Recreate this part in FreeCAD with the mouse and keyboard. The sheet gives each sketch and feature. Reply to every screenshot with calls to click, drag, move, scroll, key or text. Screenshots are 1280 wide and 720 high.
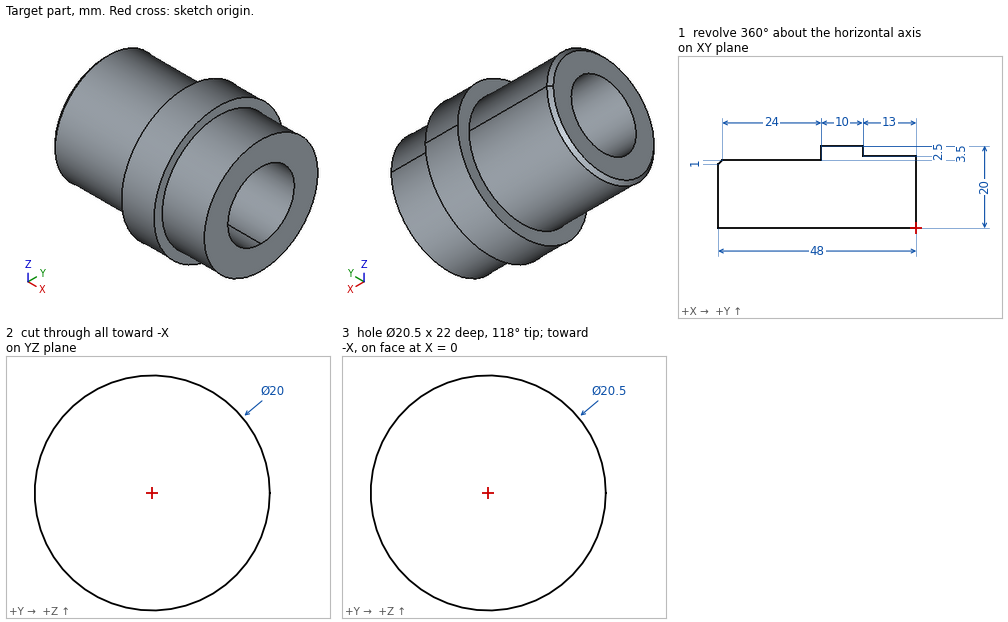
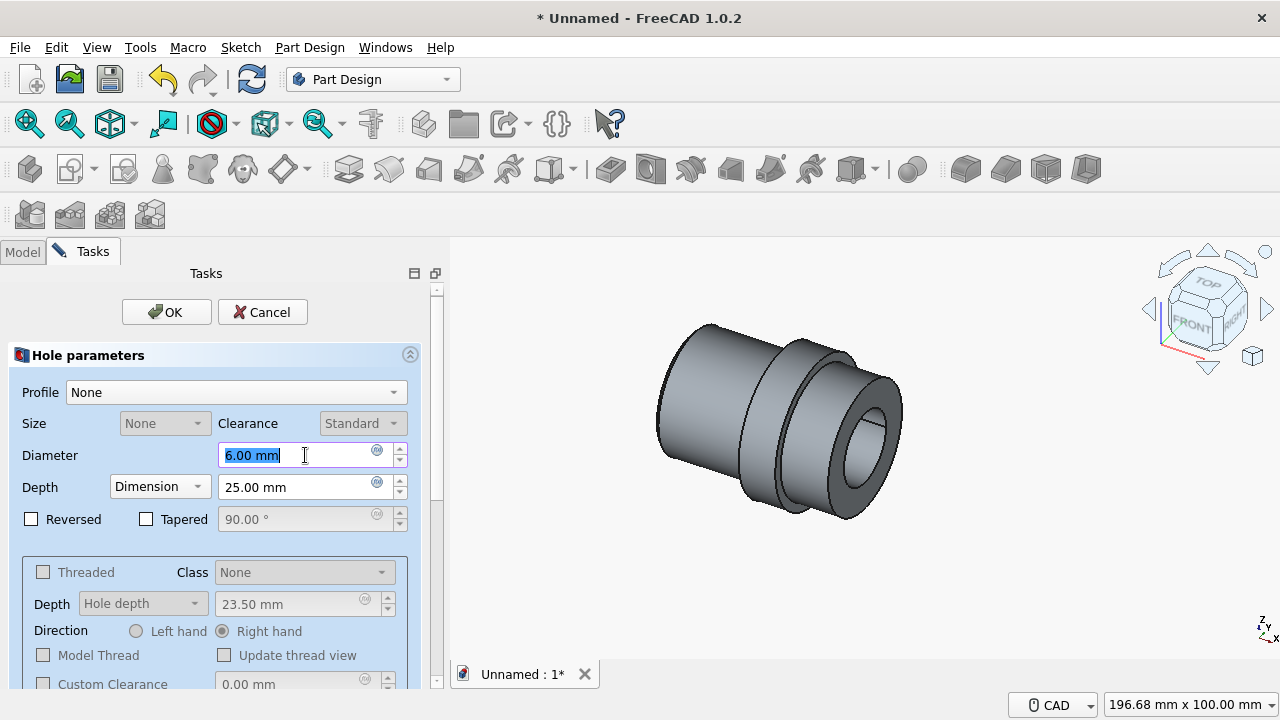
text(20.5)
key(Tab)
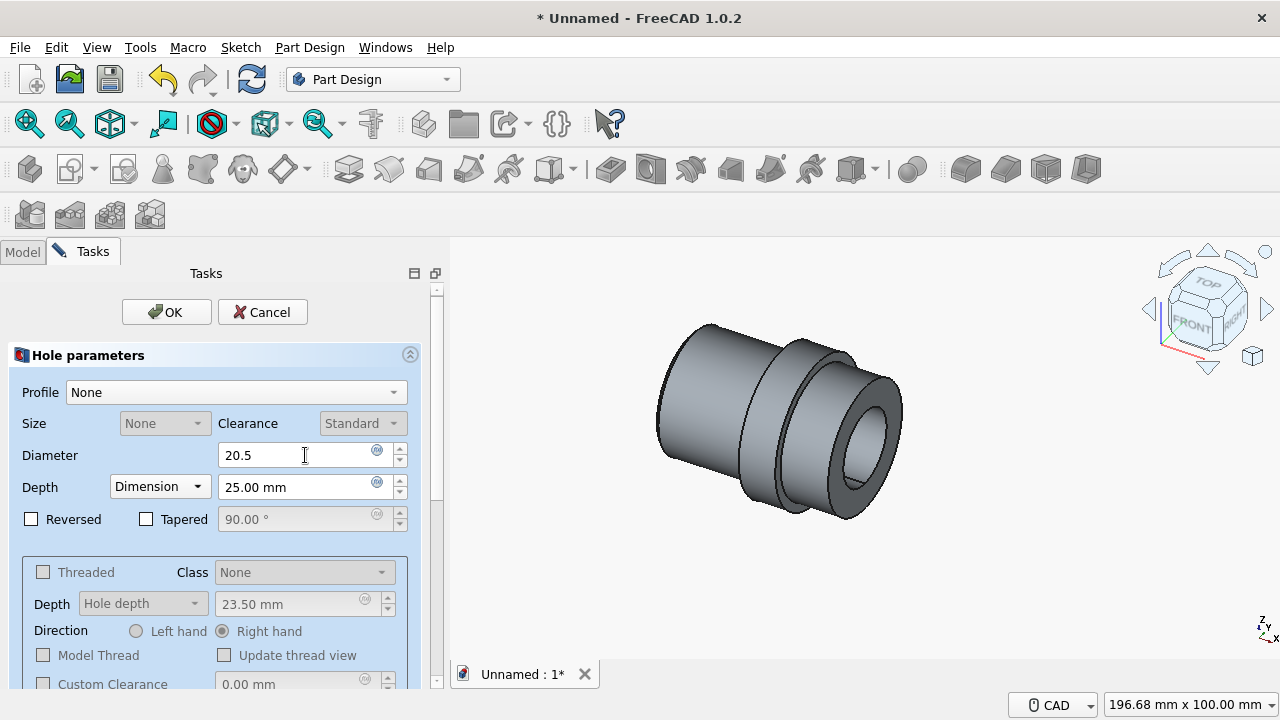
triple_click(305, 487)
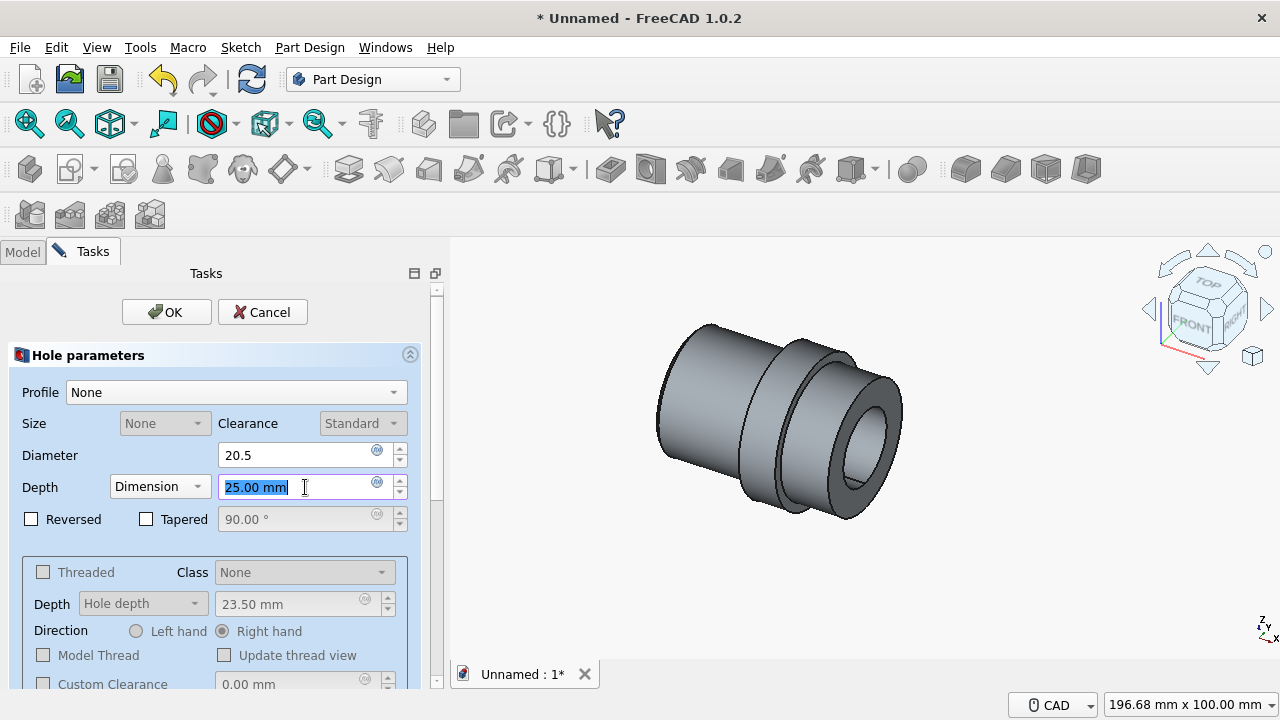
text(22)
key(Tab)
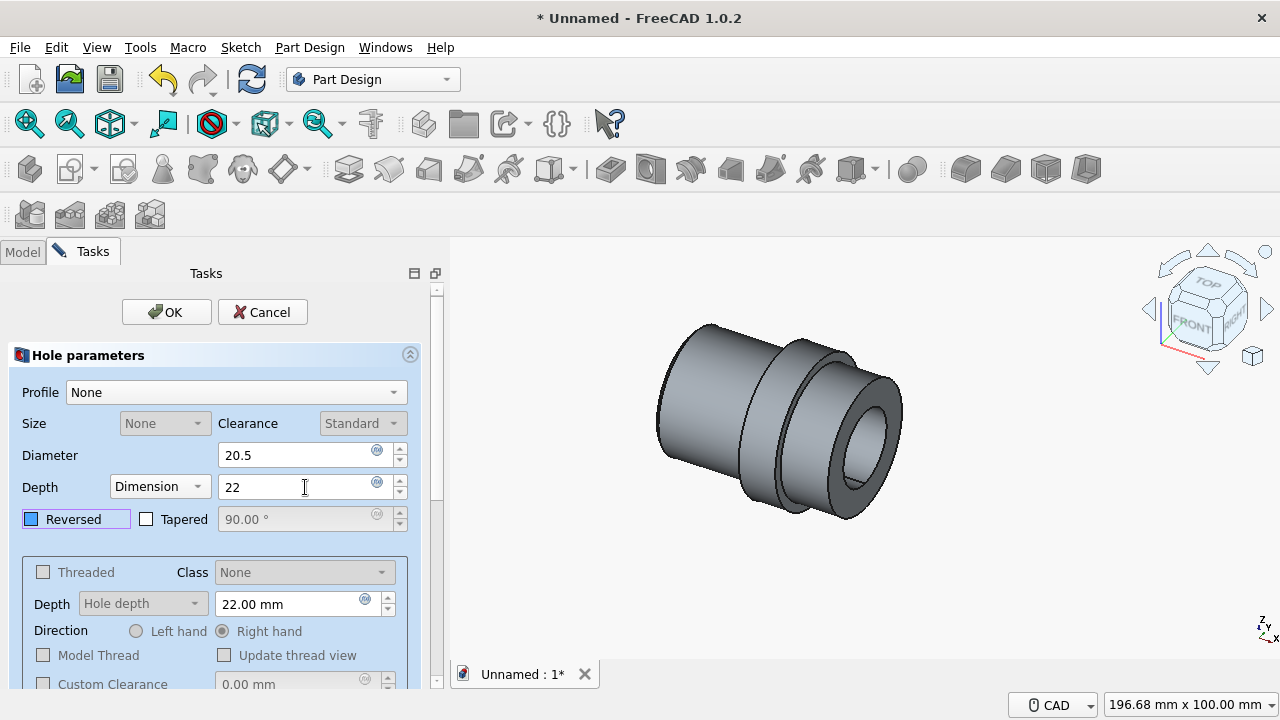
click(167, 312)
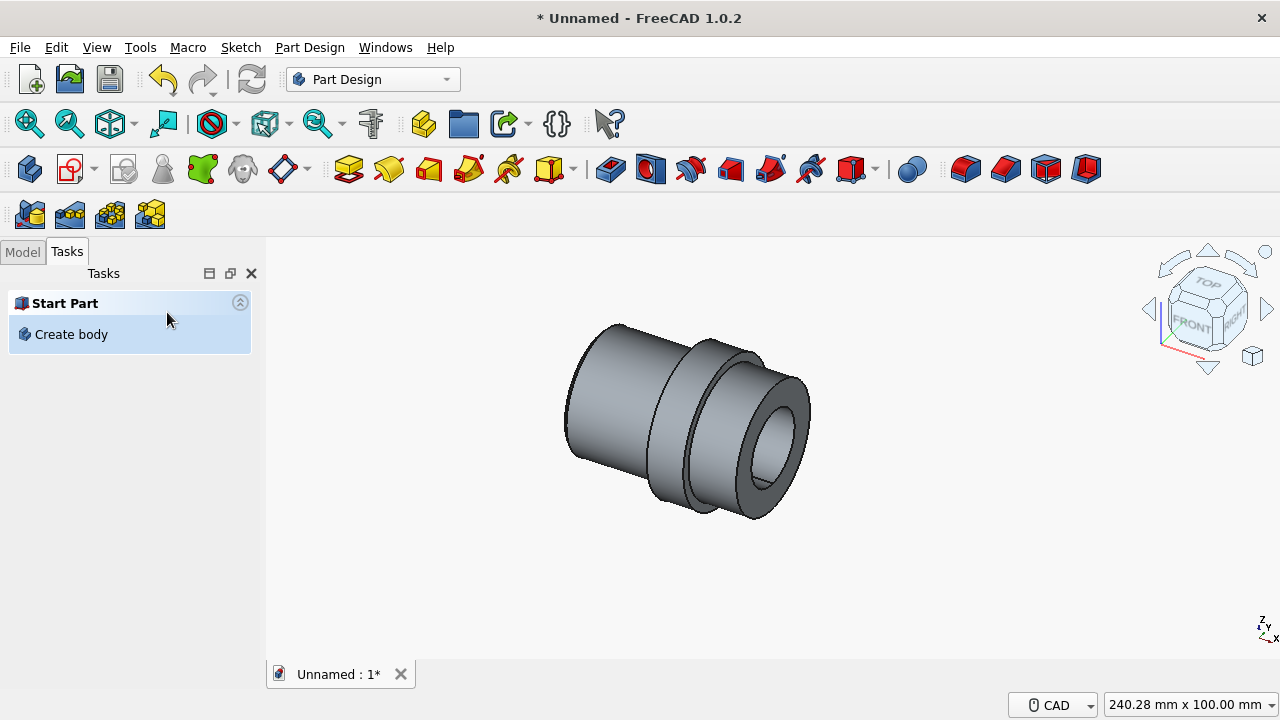
key(0)